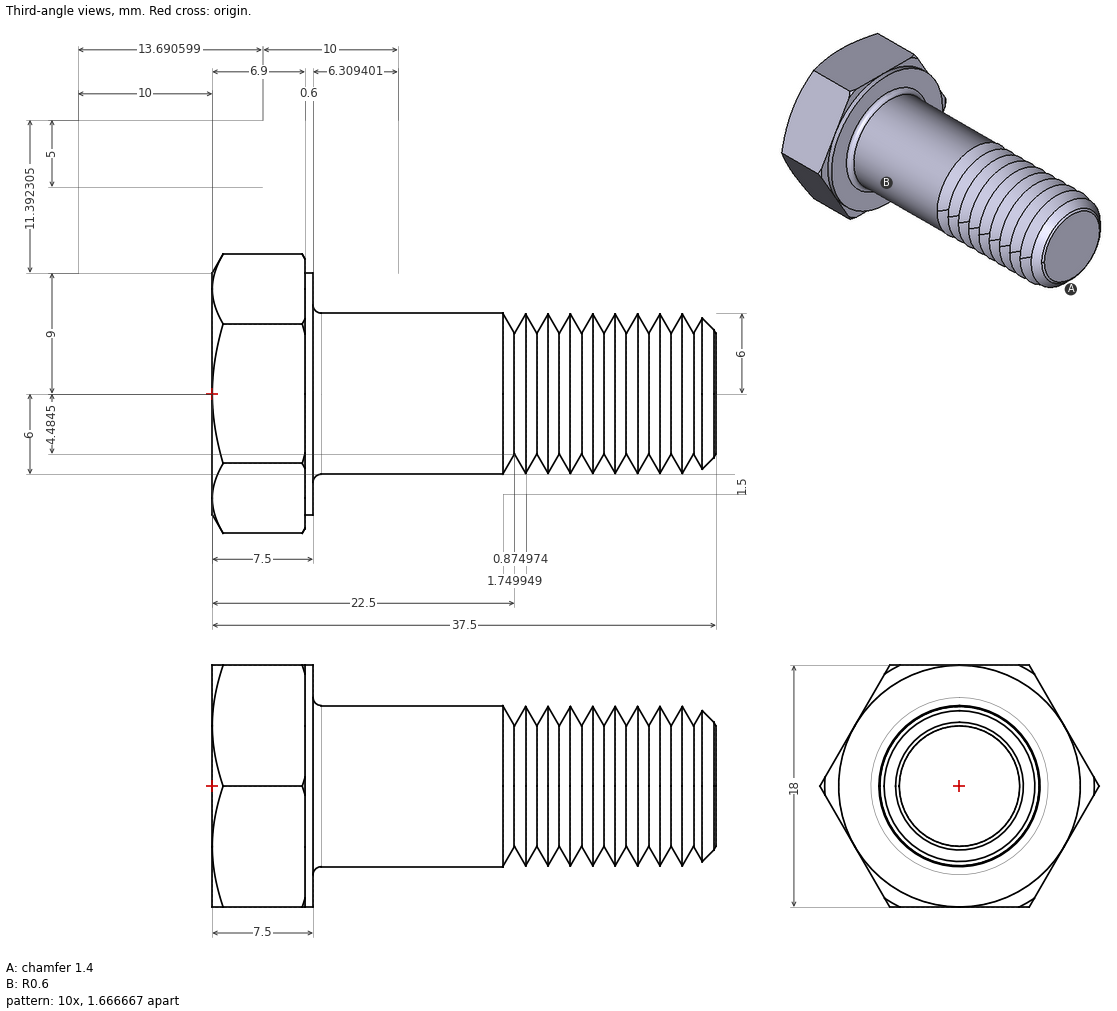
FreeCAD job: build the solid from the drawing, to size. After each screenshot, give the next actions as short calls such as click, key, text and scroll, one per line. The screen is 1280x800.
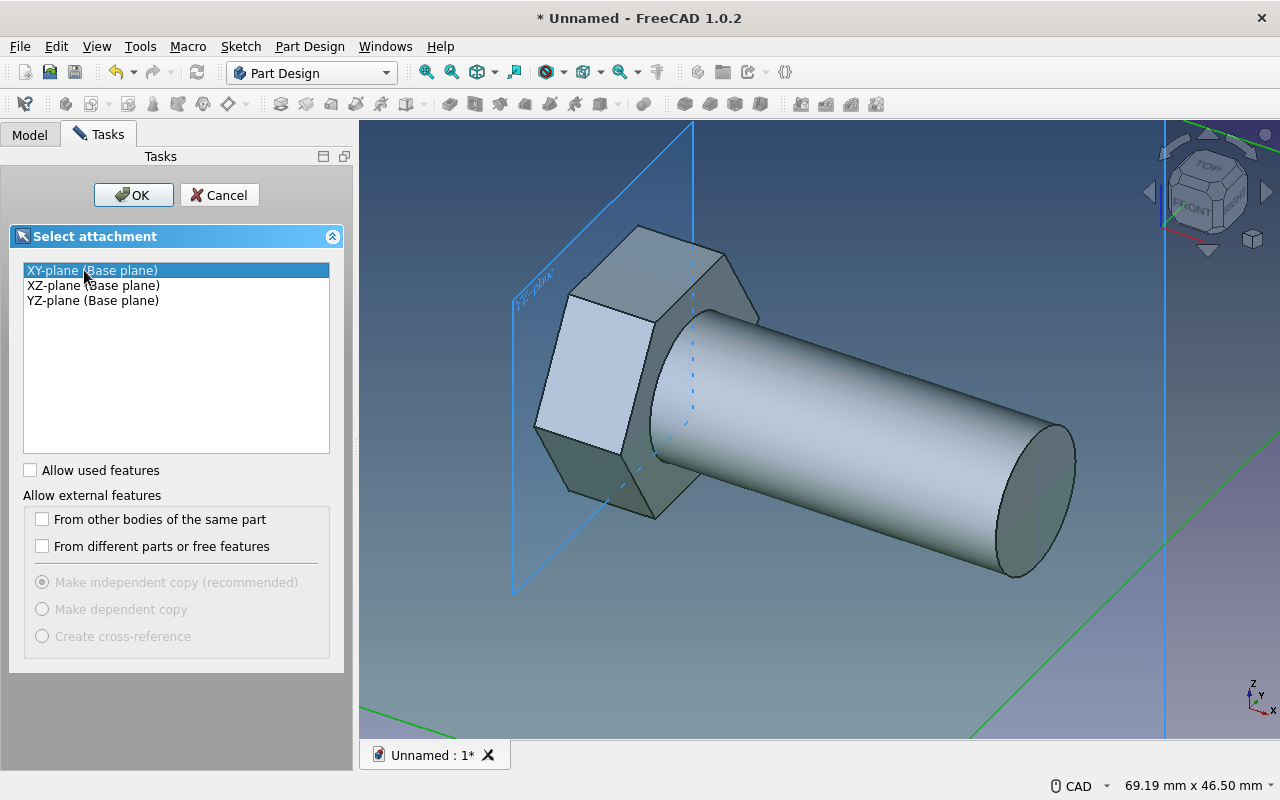
click(134, 195)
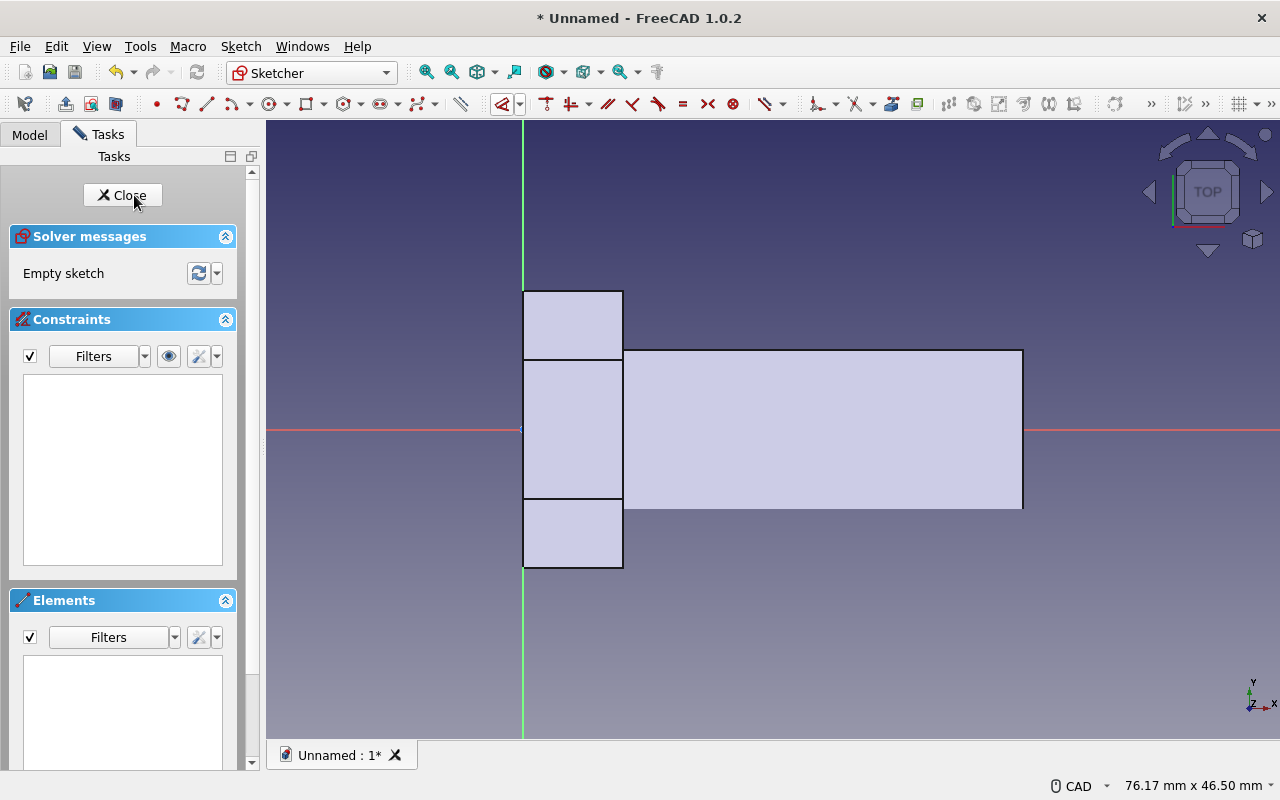
click(116, 104)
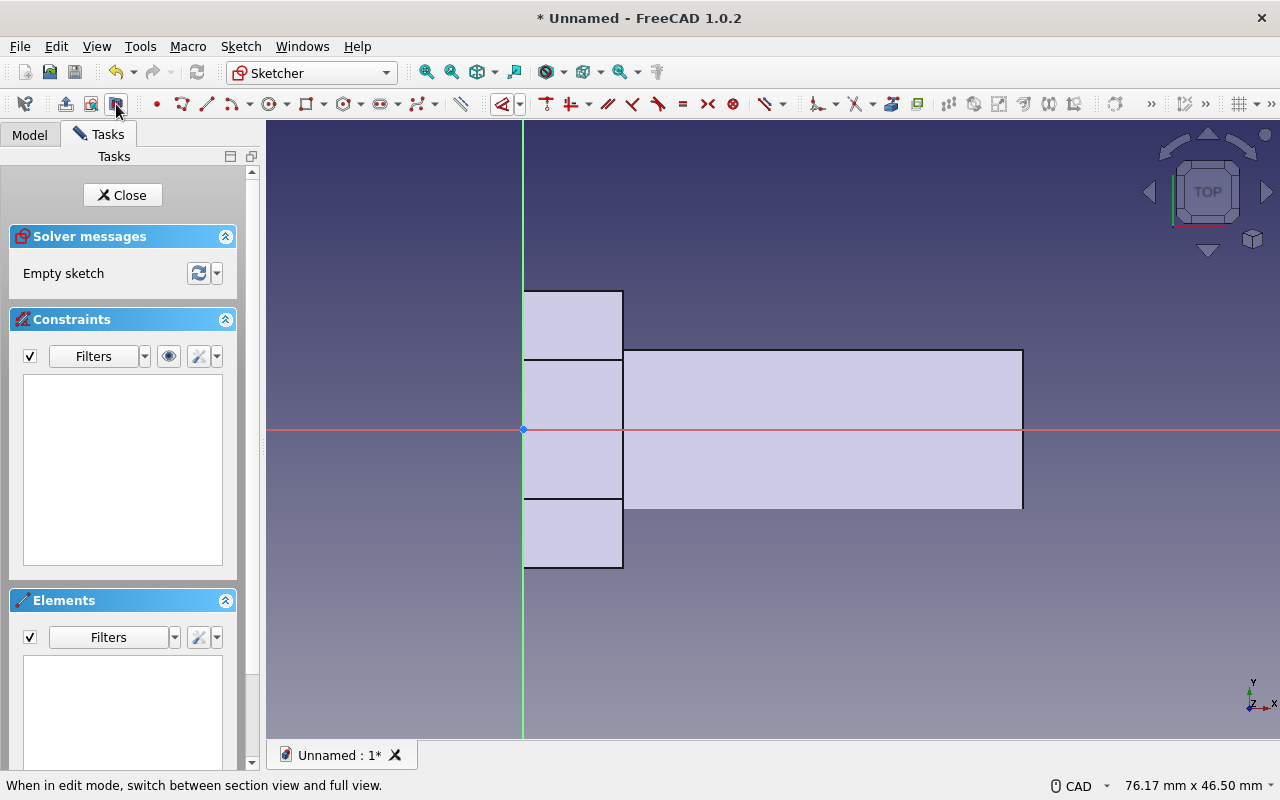
scroll(1115, 711, down, 1)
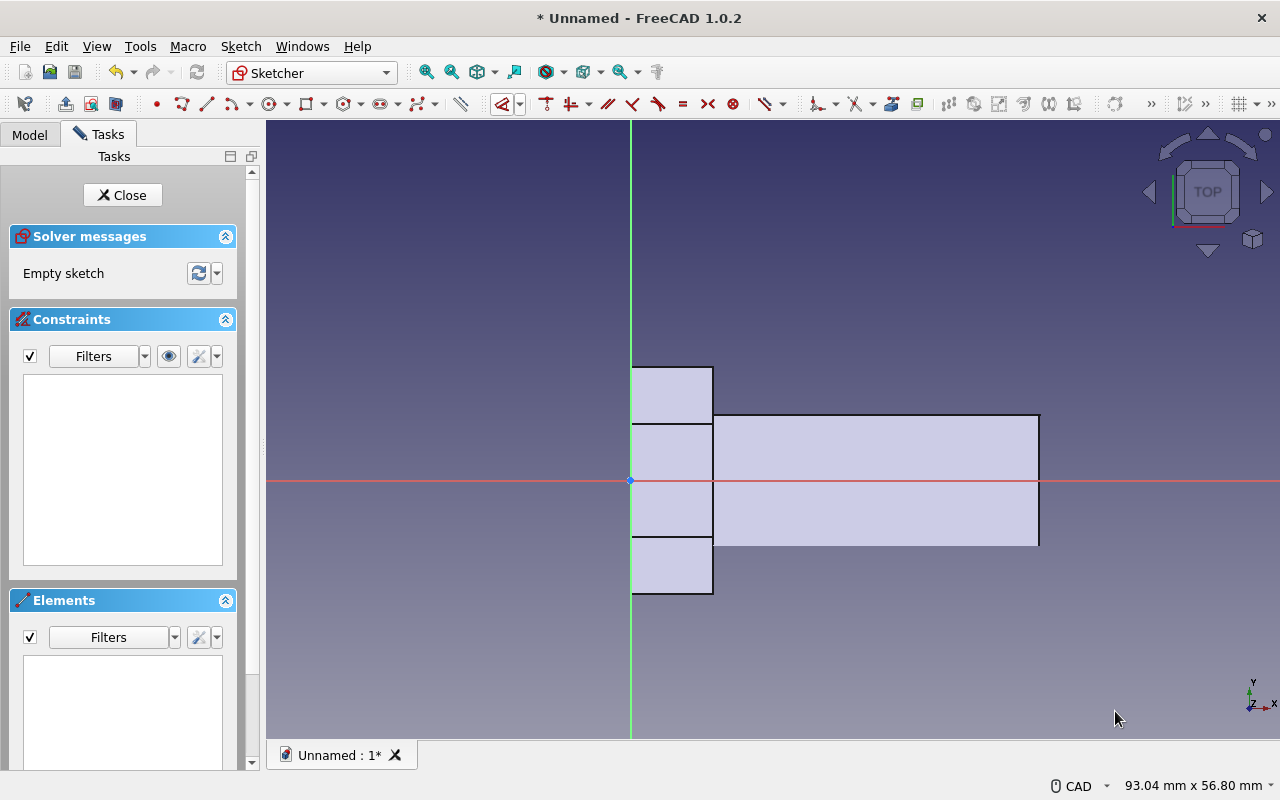
scroll(465, 297, up, 3)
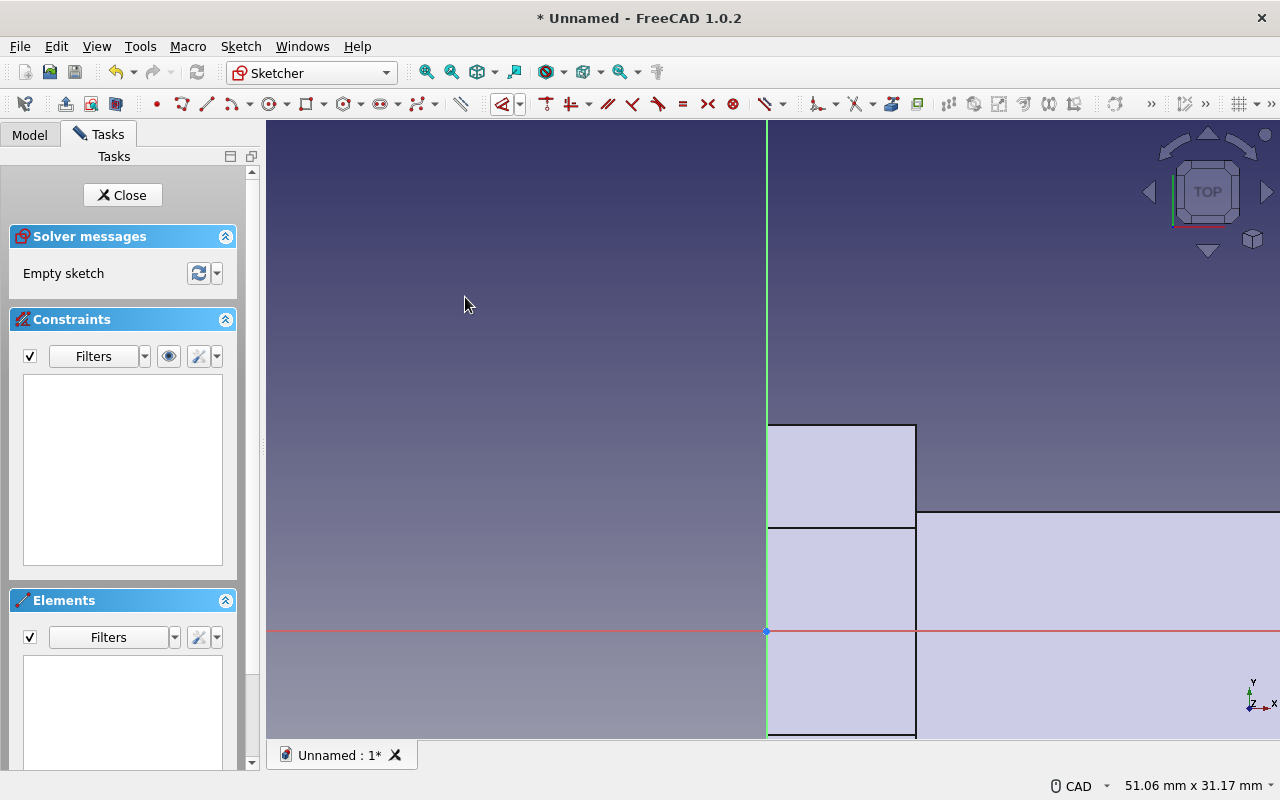
click(182, 104)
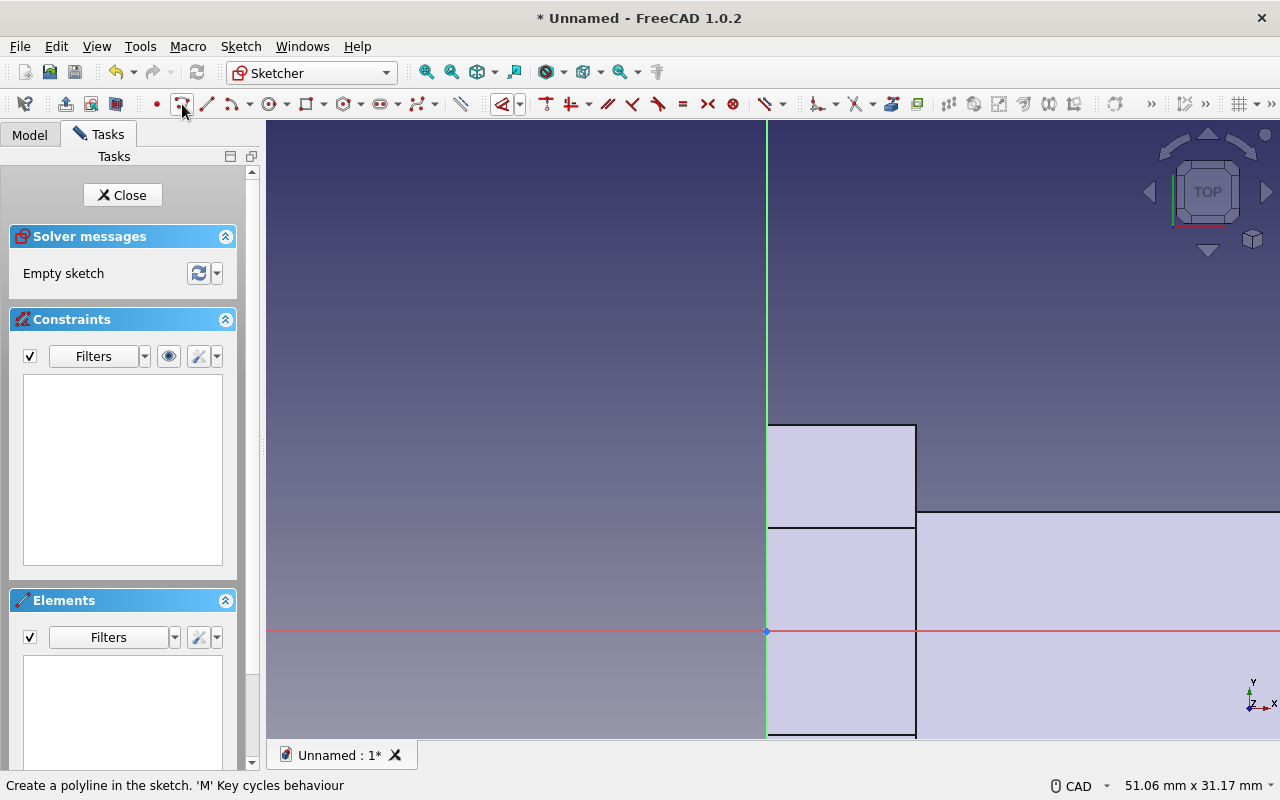
click(767, 453)
click(840, 326)
click(840, 227)
click(568, 227)
click(568, 453)
click(767, 454)
key(Escape)
key(Escape)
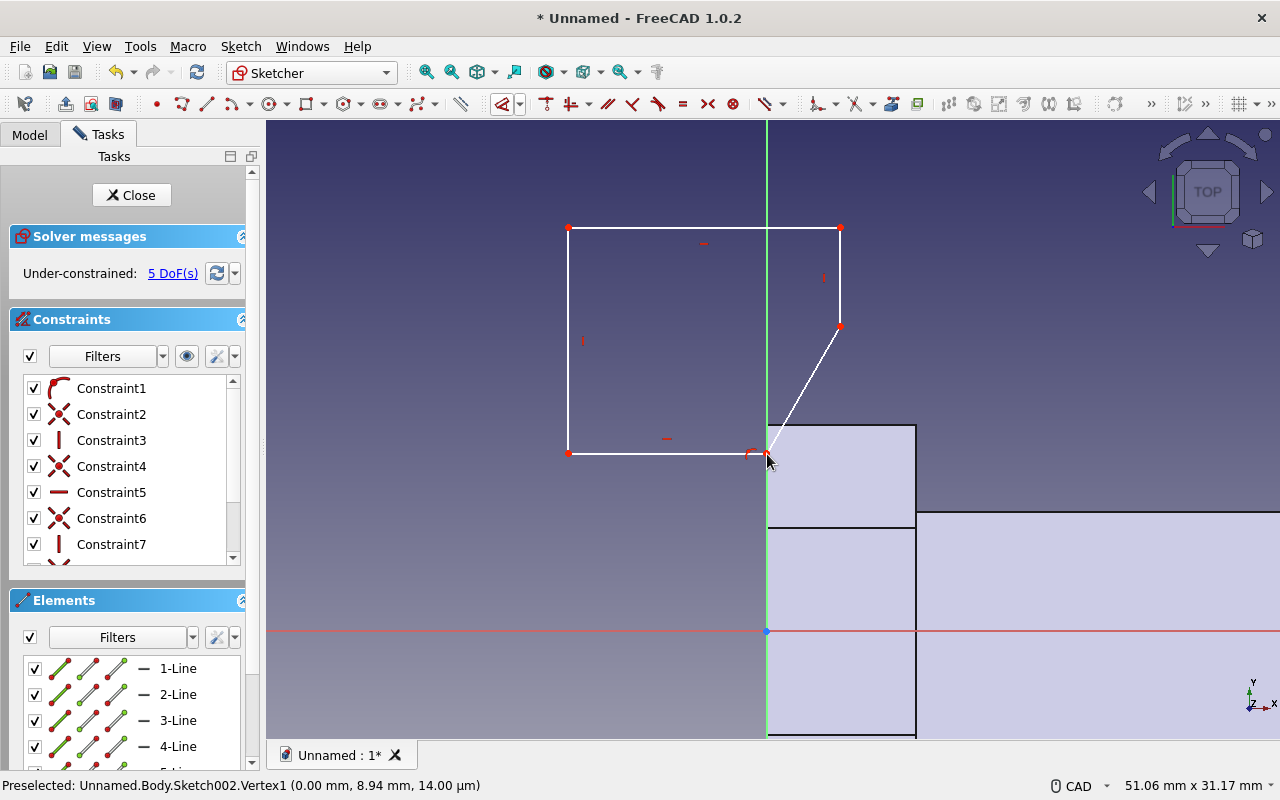
click(840, 297)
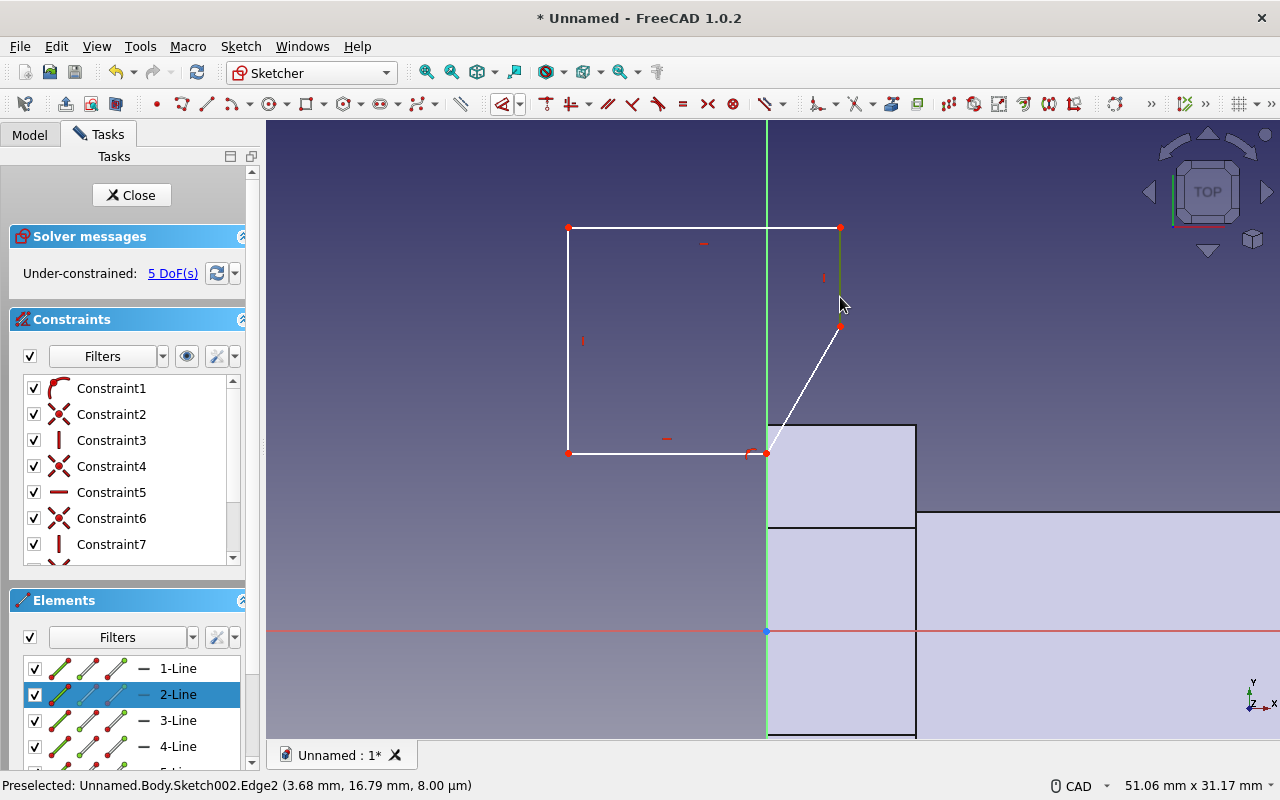
click(520, 104)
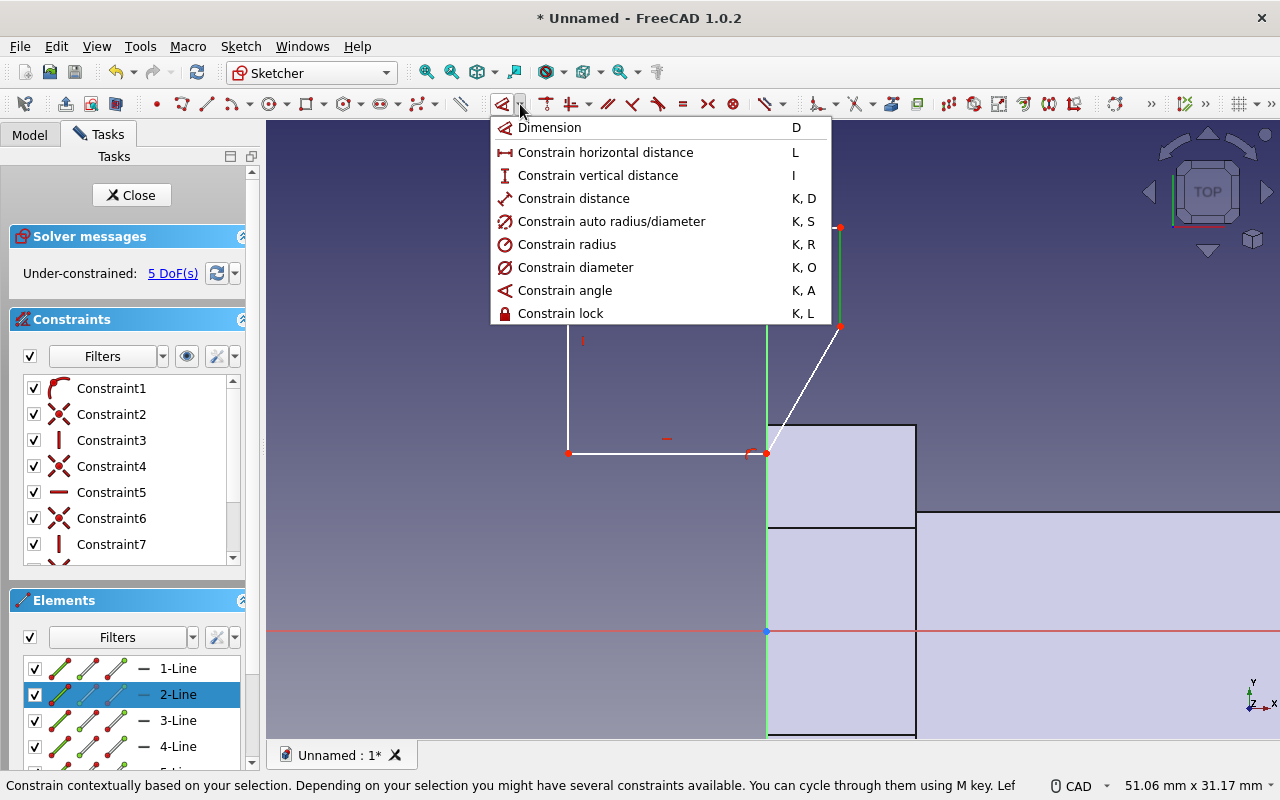
click(661, 176)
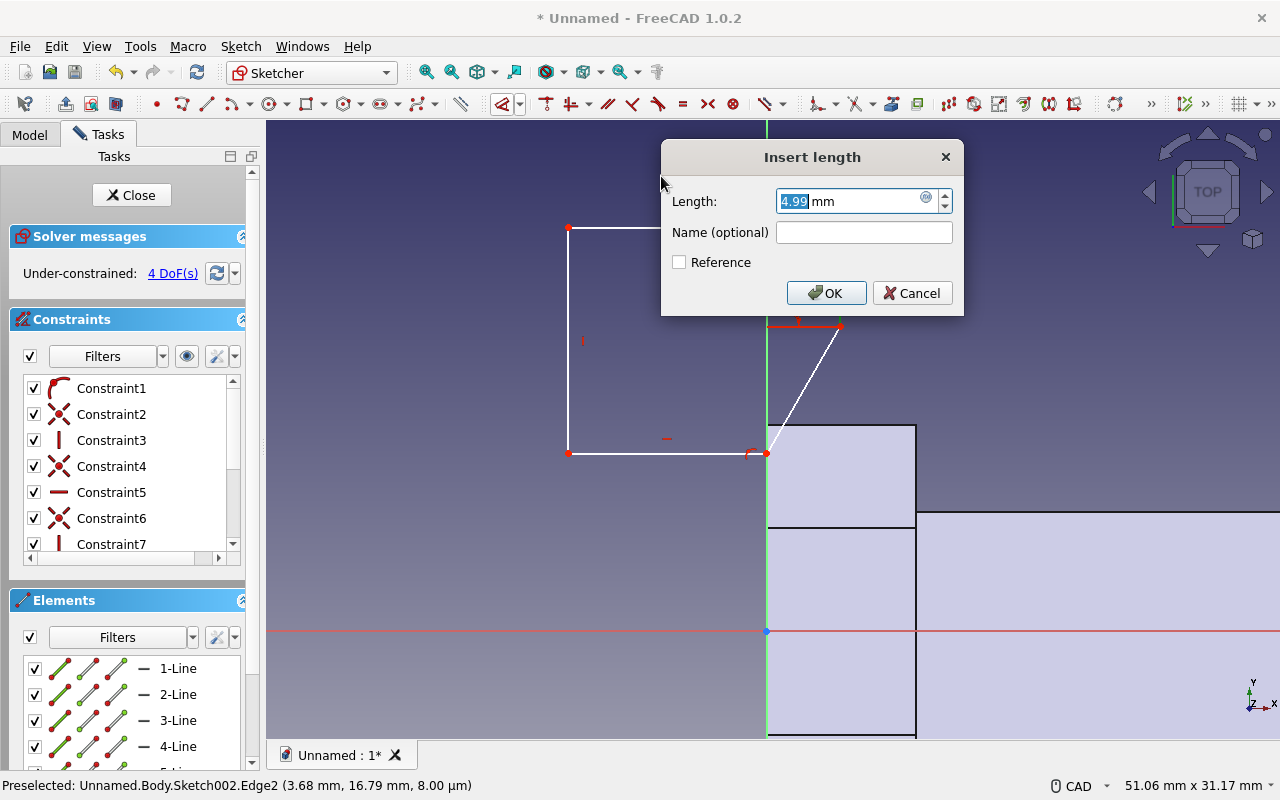
text(5)
key(Return)